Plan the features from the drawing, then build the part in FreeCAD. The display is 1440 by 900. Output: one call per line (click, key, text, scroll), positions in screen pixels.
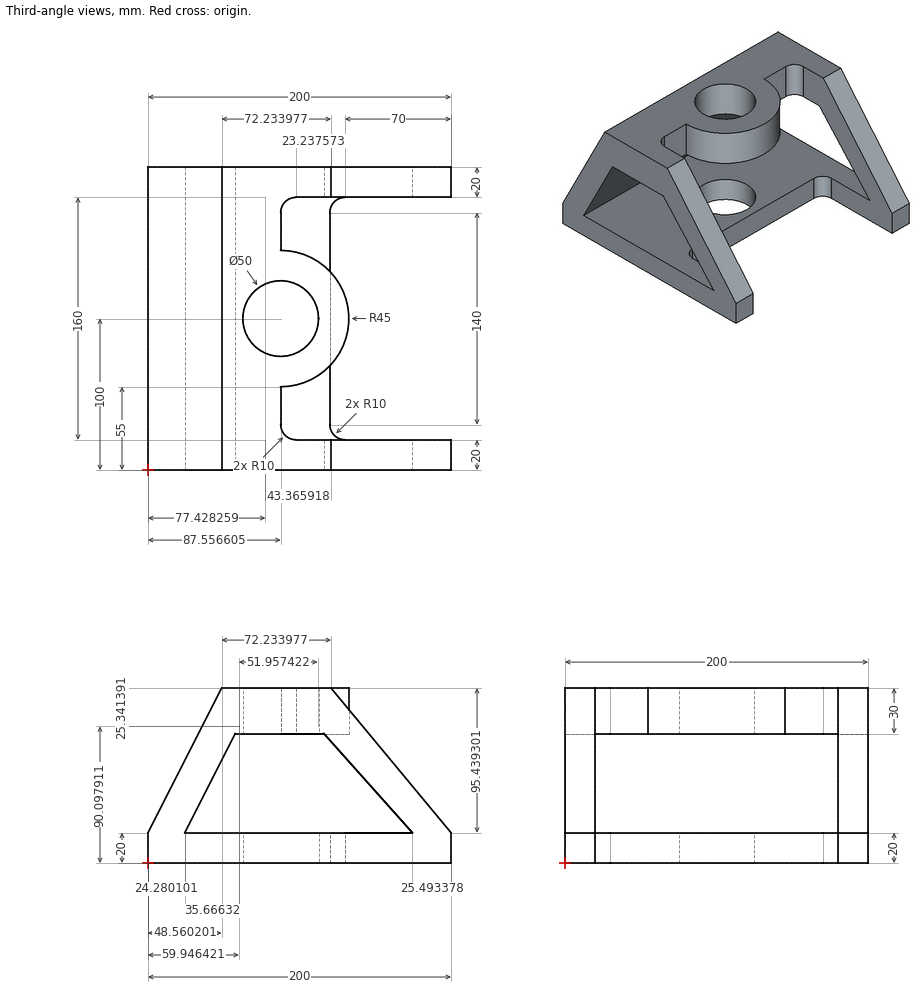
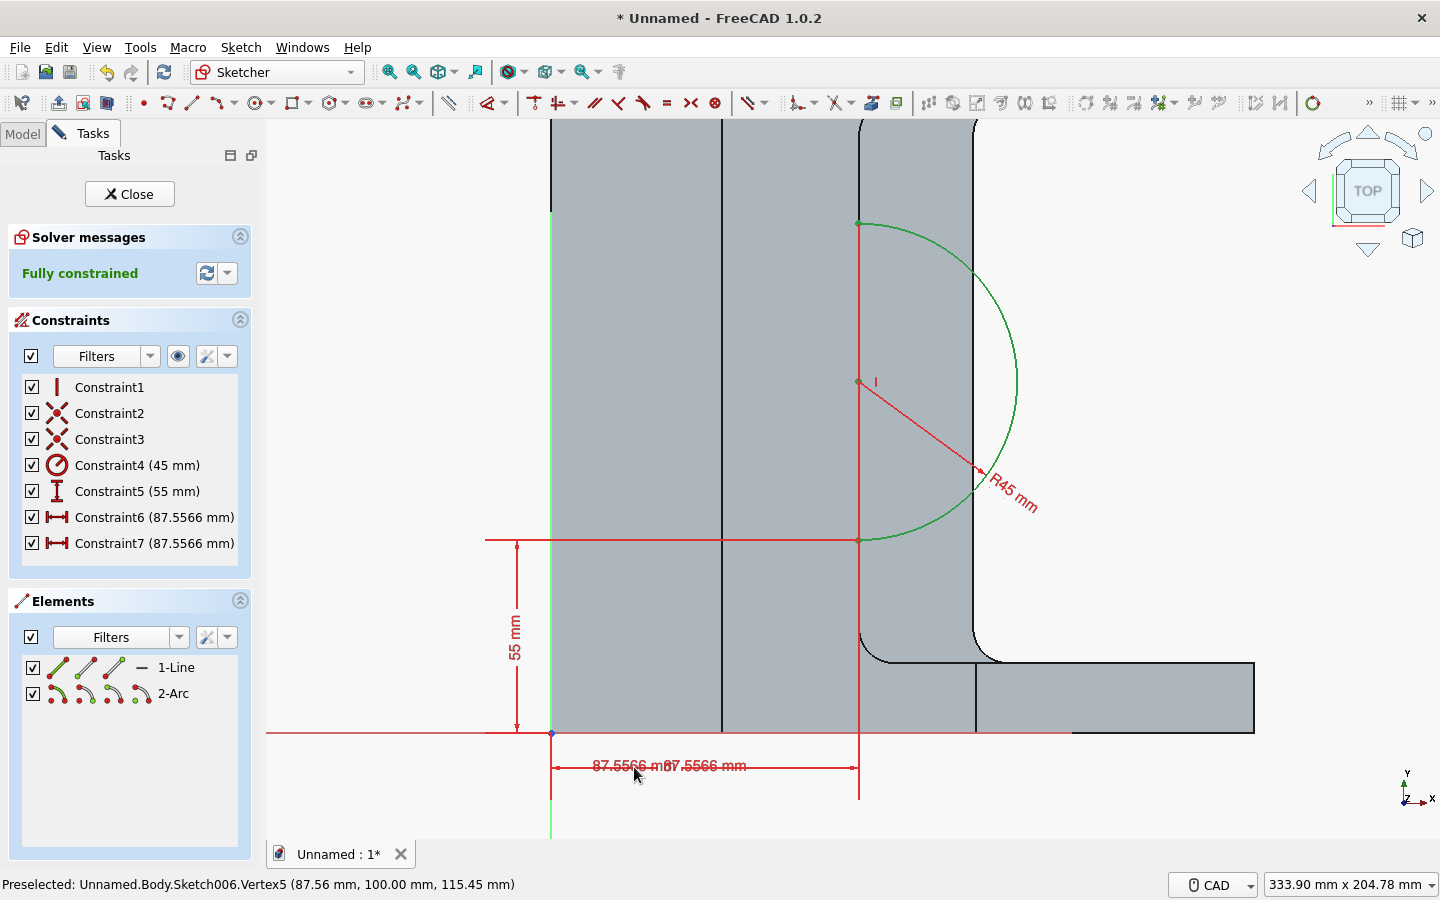
click(130, 194)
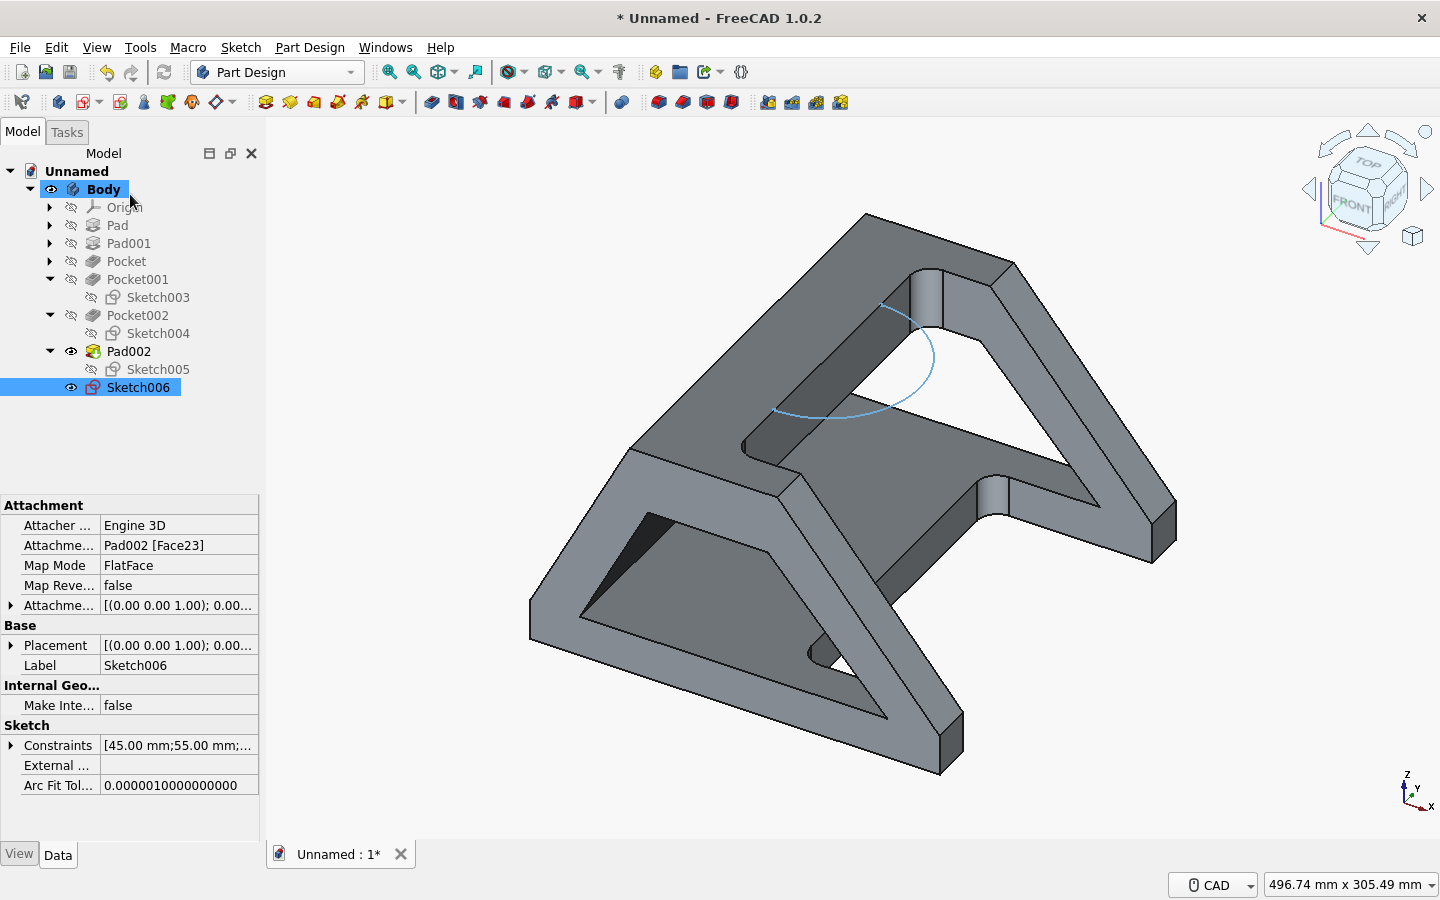
click(266, 102)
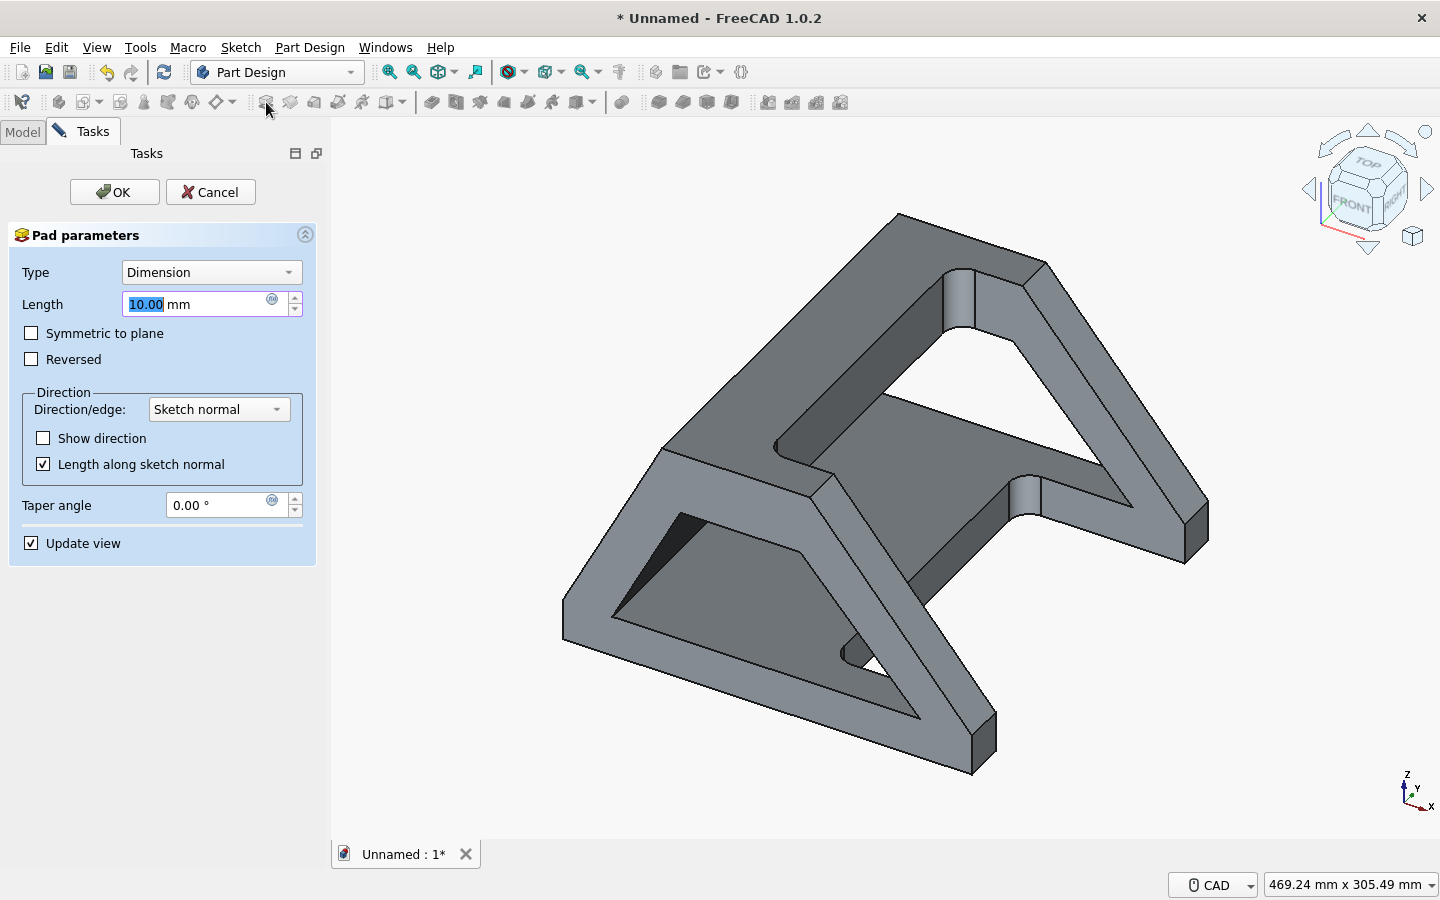
text(30)
key(Tab)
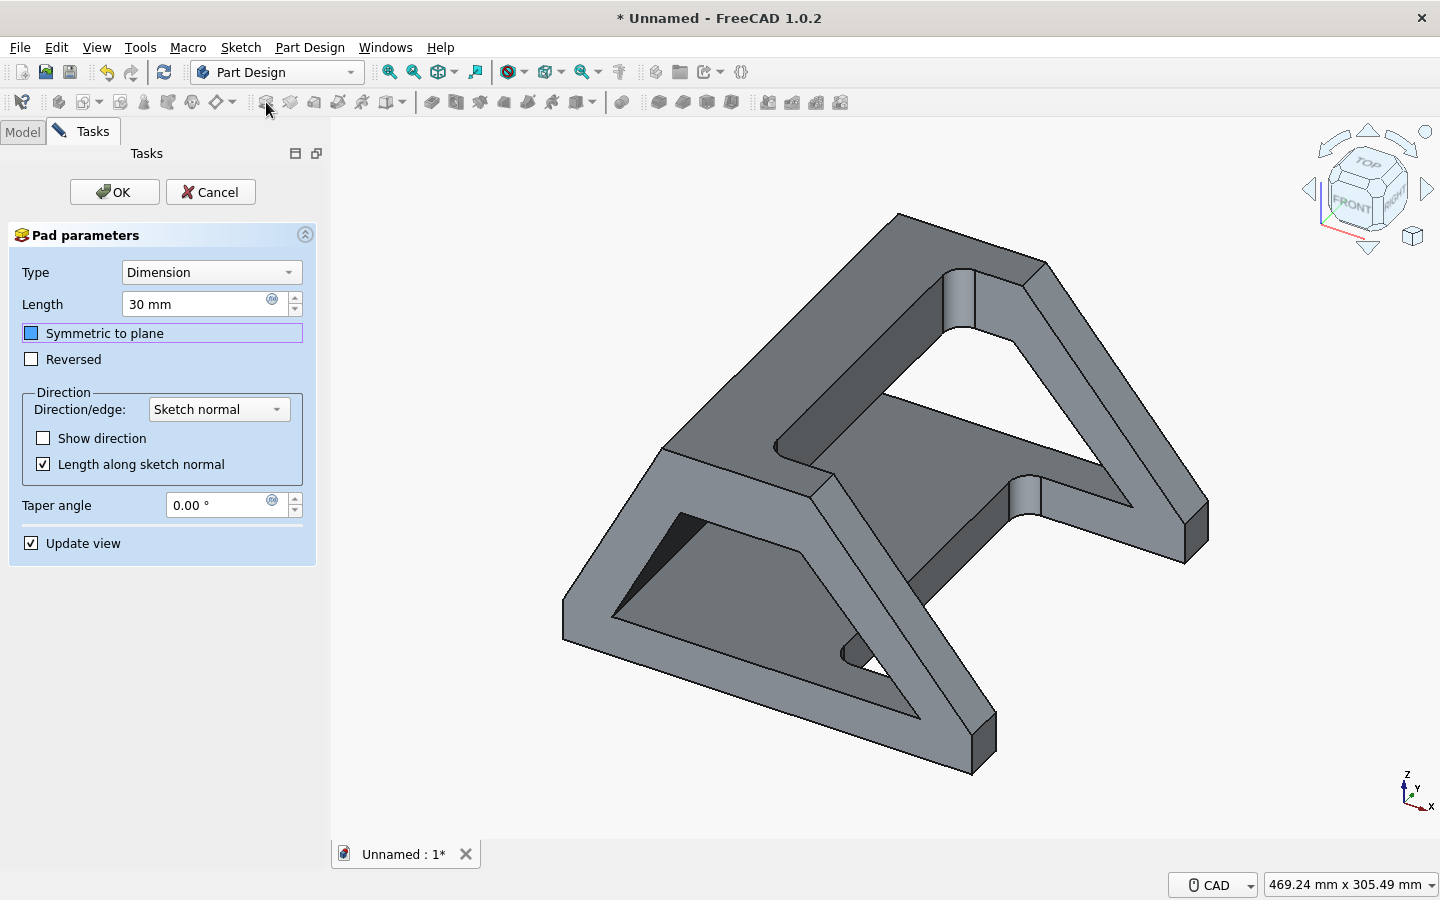
click(30, 359)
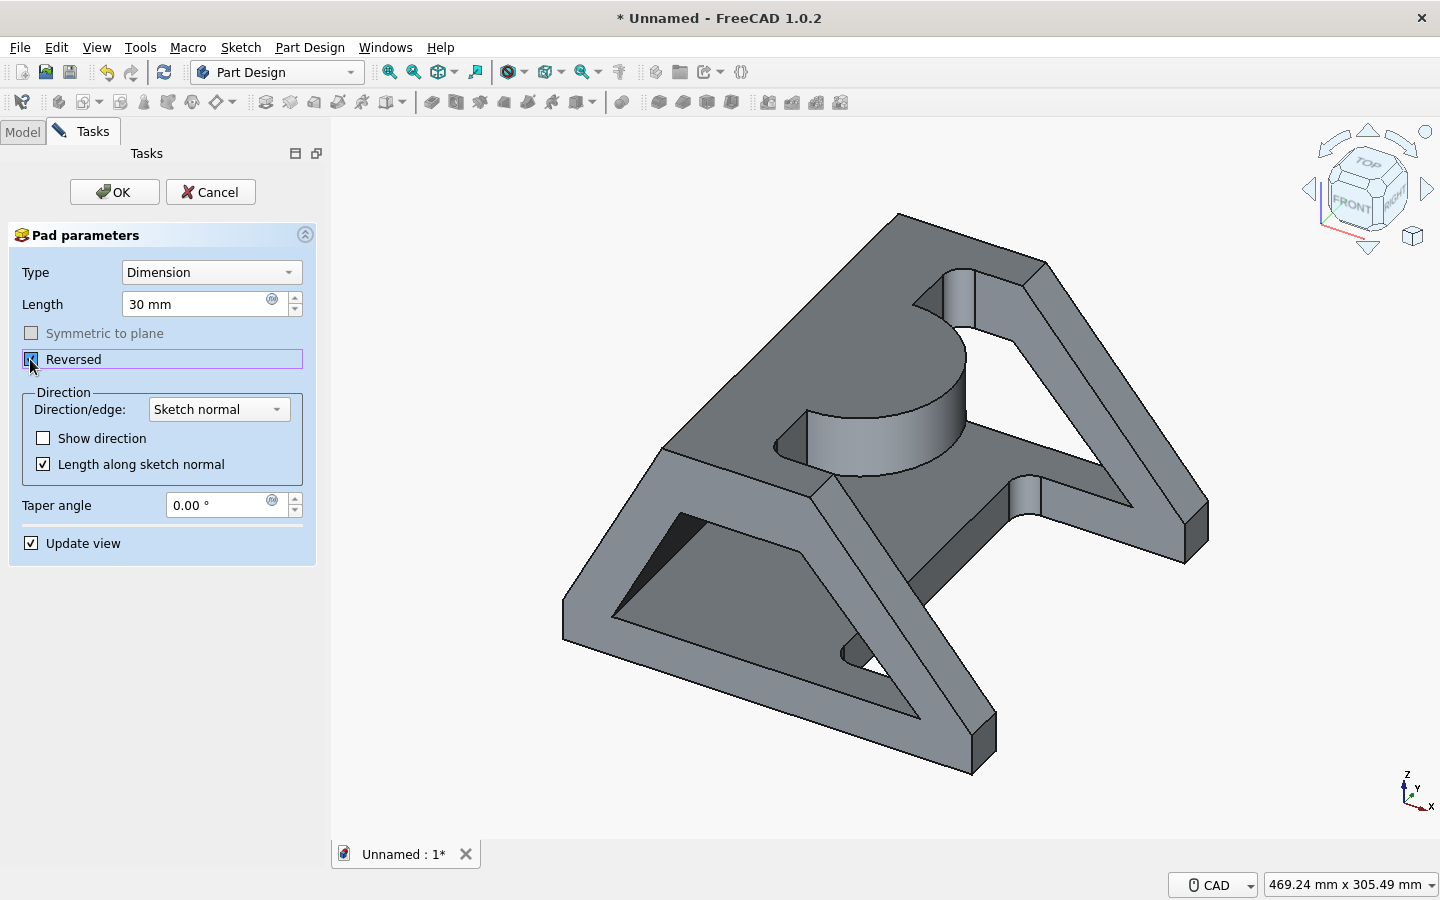
click(115, 192)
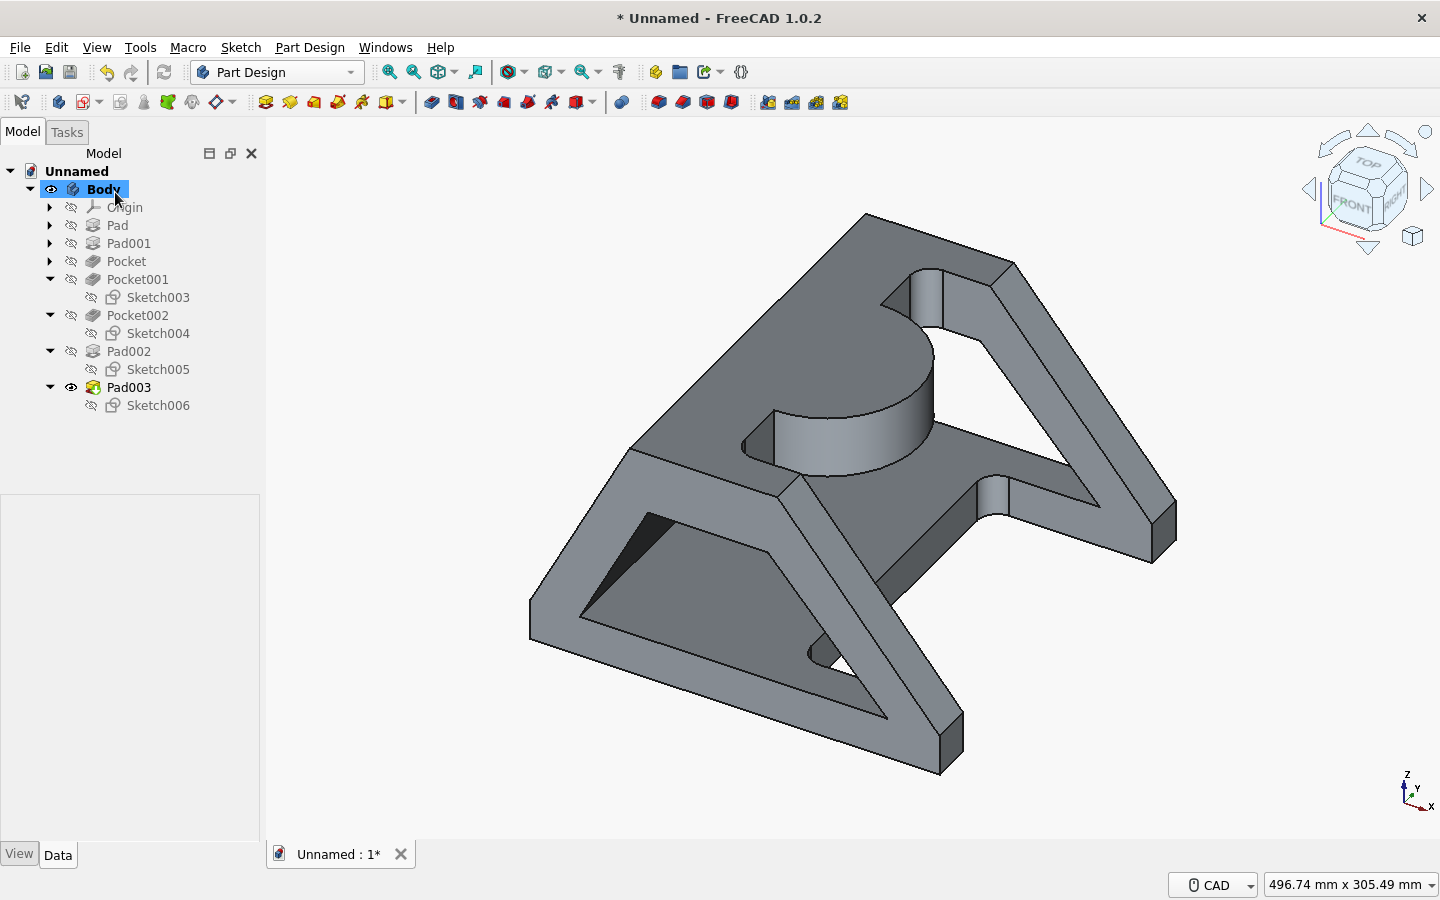
click(834, 359)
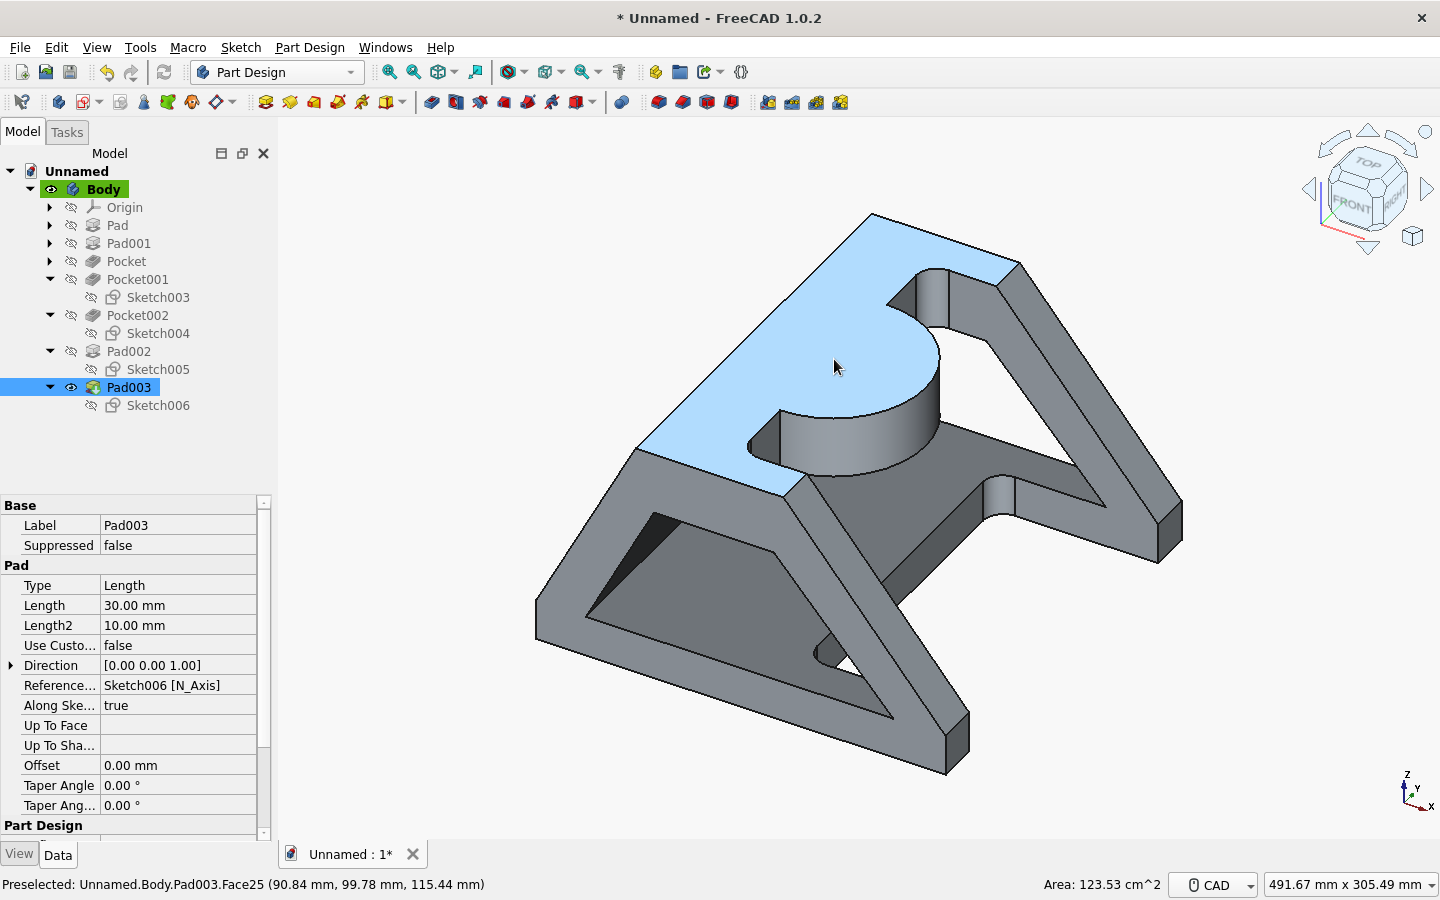
click(84, 102)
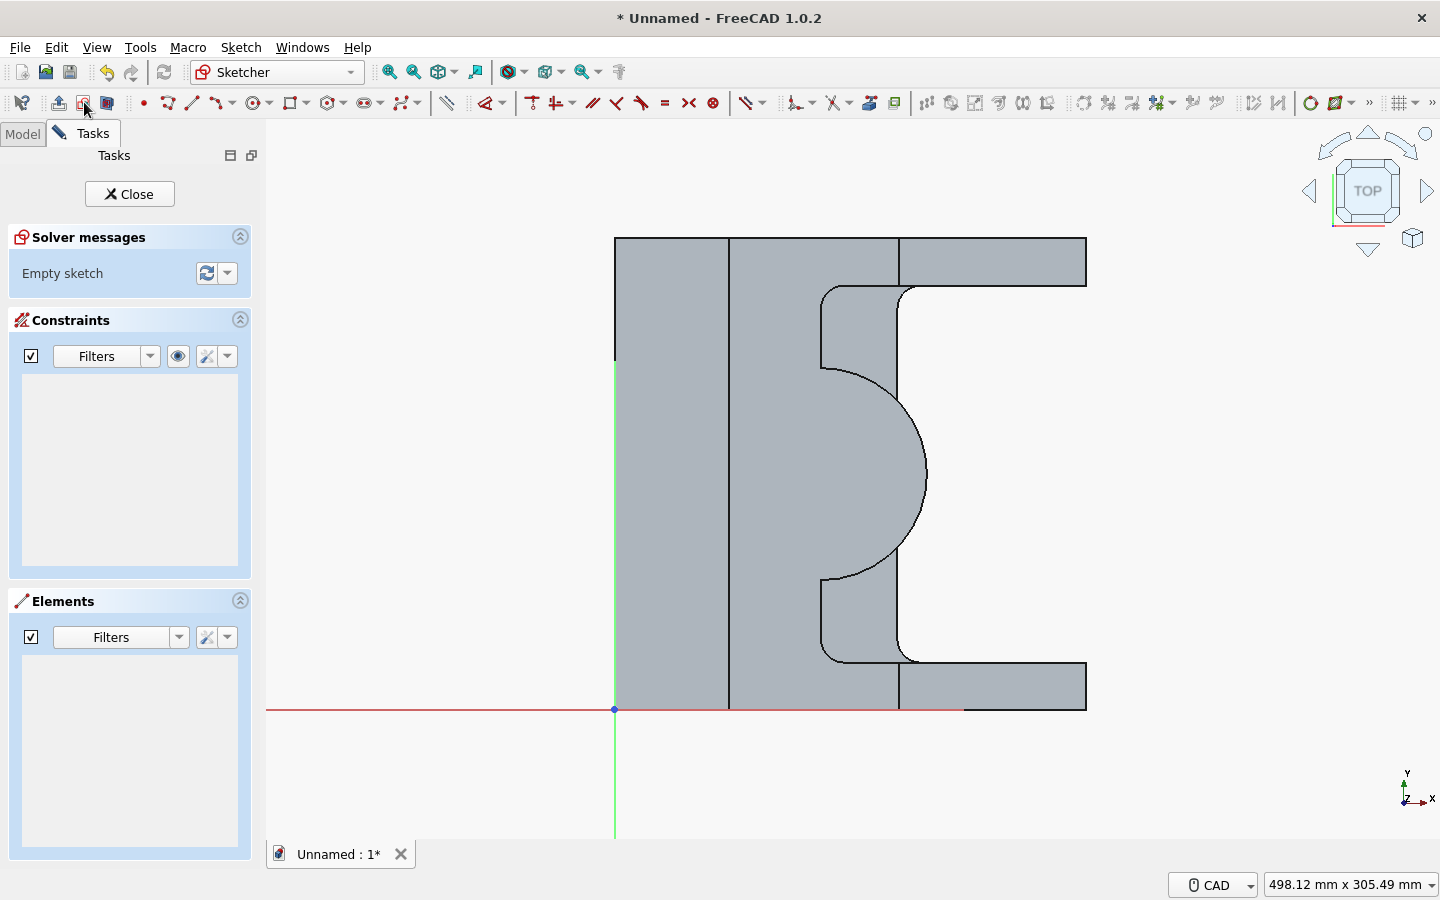
scroll(833, 473, up, 7)